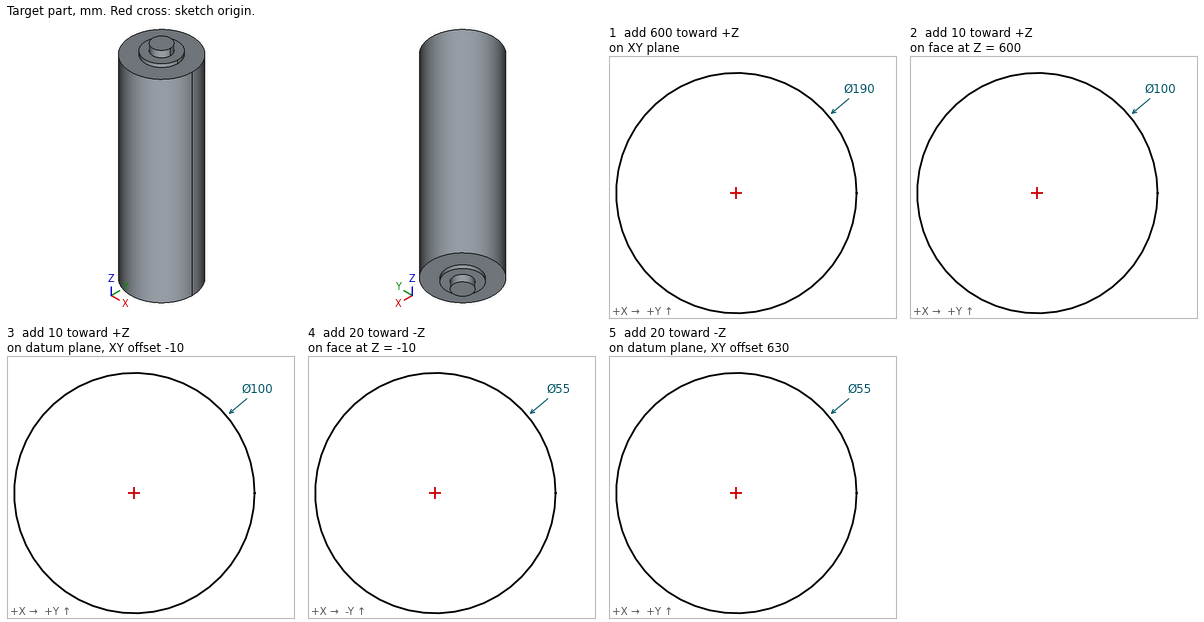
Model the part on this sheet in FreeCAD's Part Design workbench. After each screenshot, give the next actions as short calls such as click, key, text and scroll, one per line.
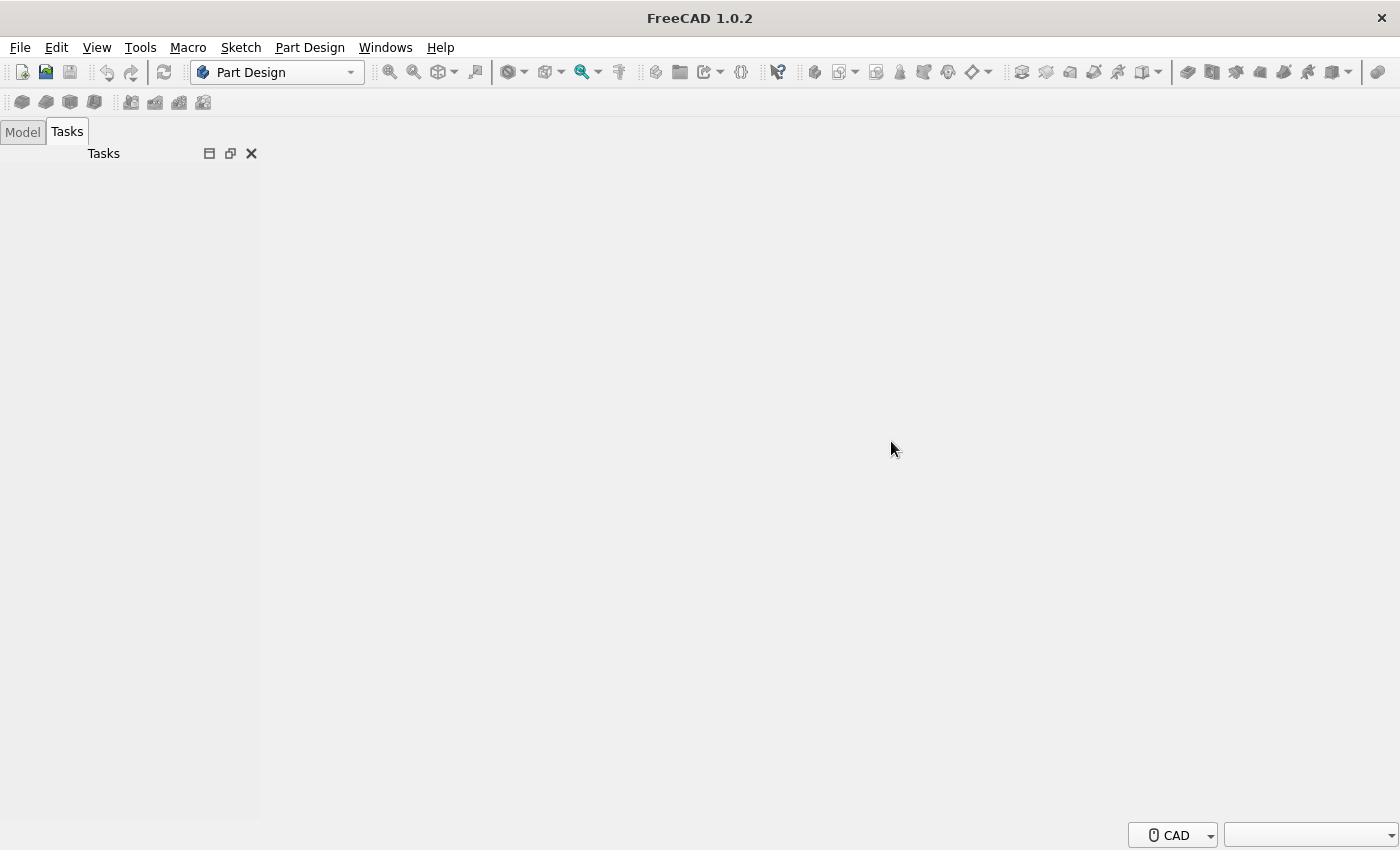
click(22, 72)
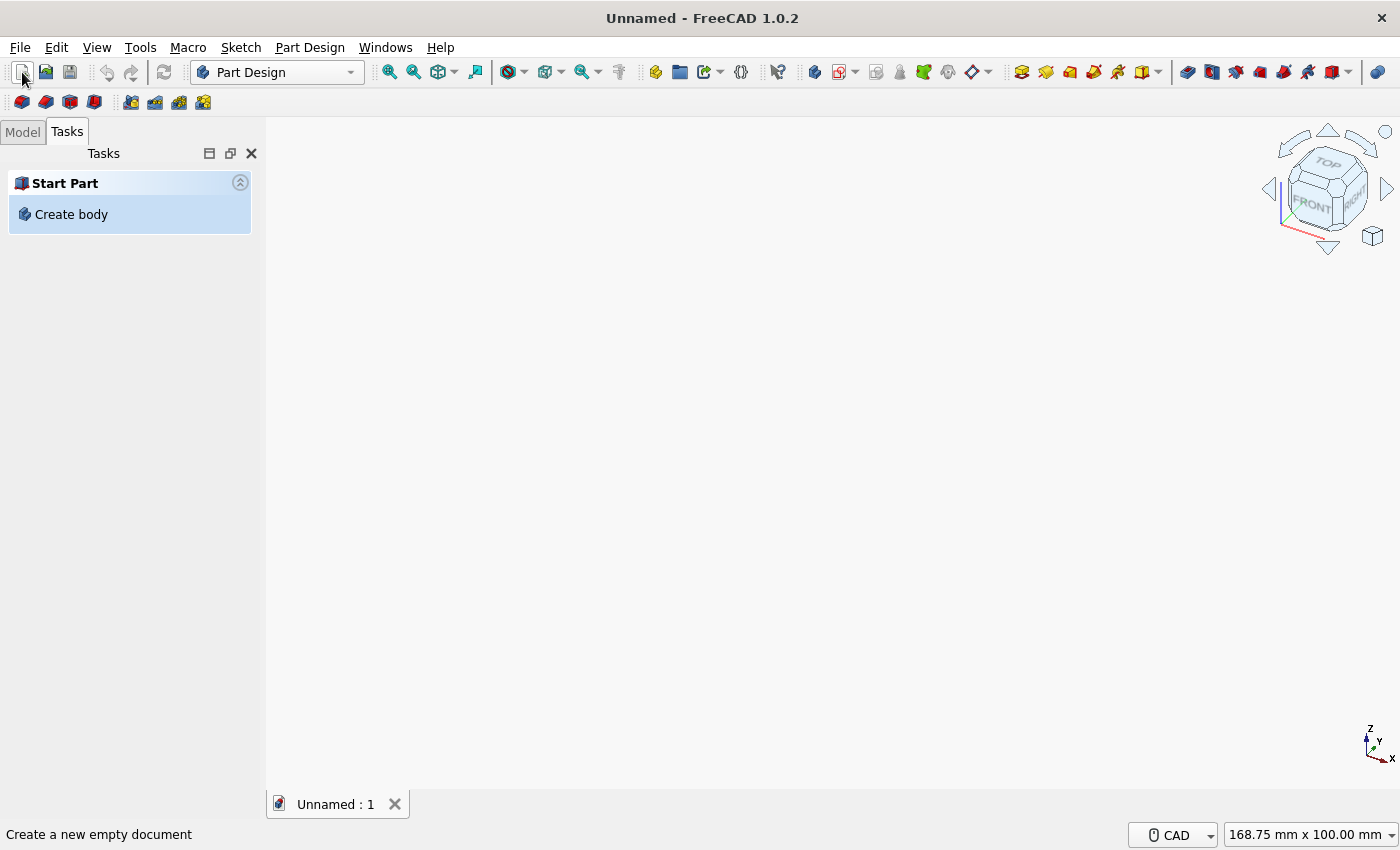
click(840, 72)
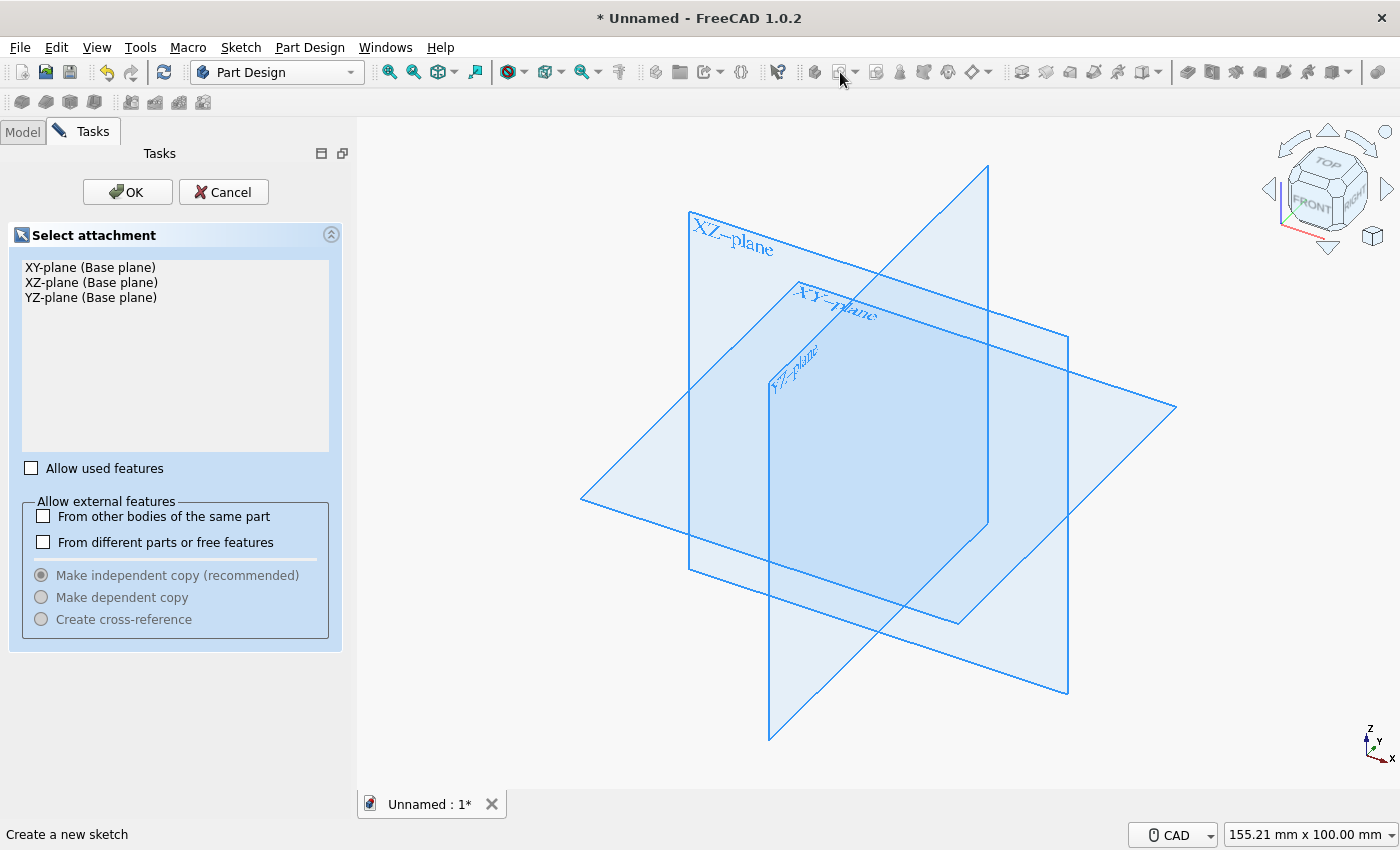
click(82, 268)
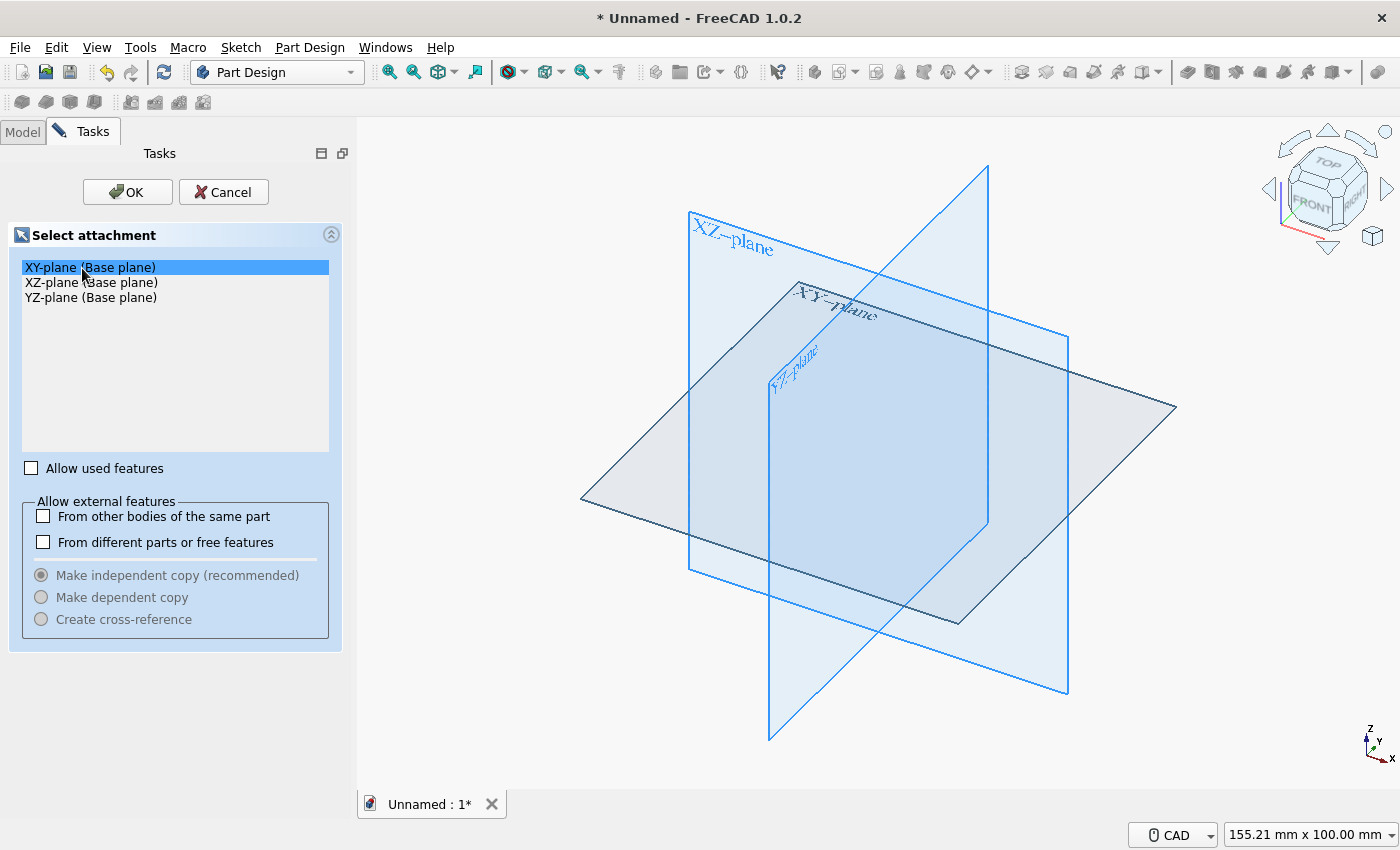
click(128, 192)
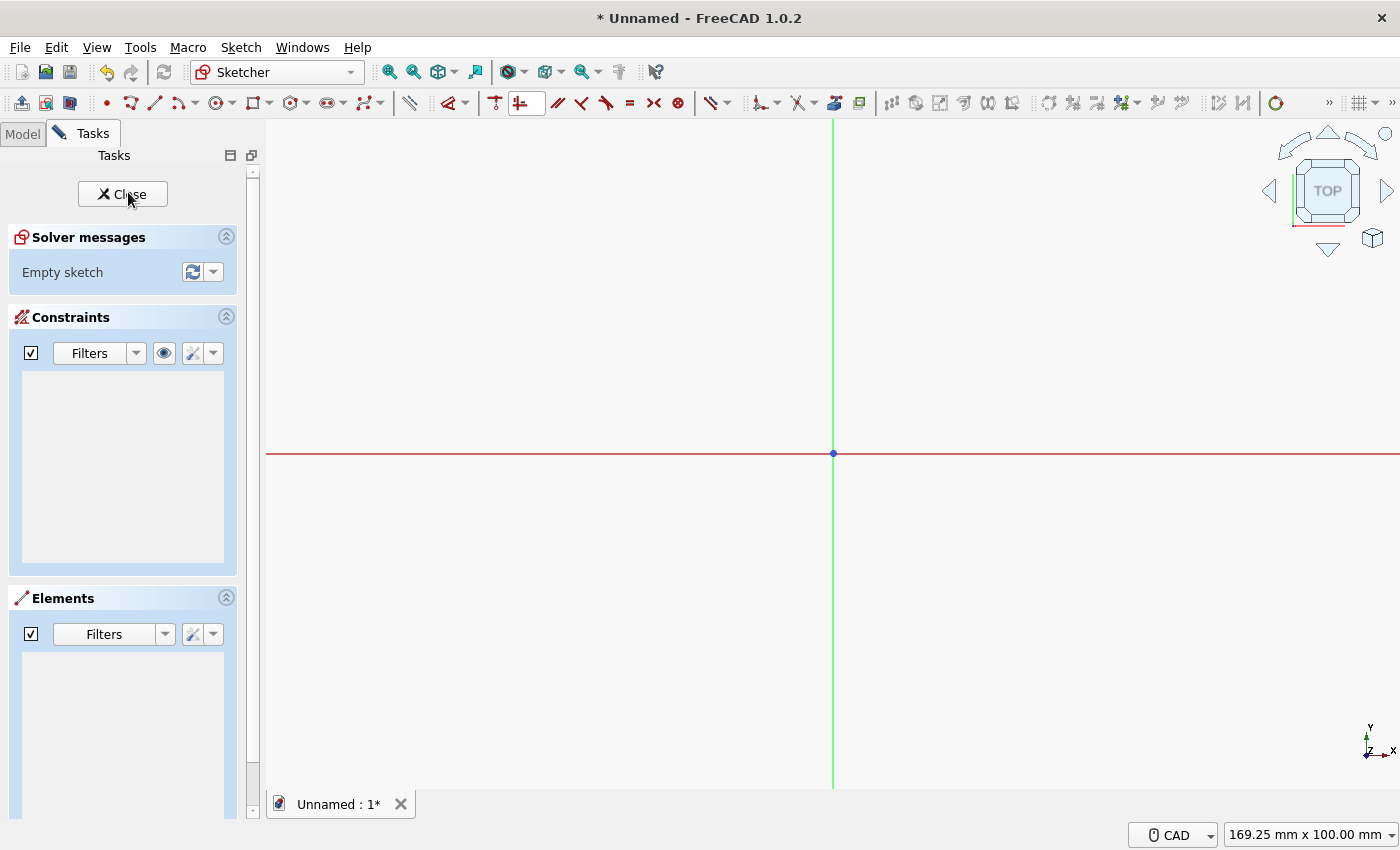
scroll(725, 454, down, 5)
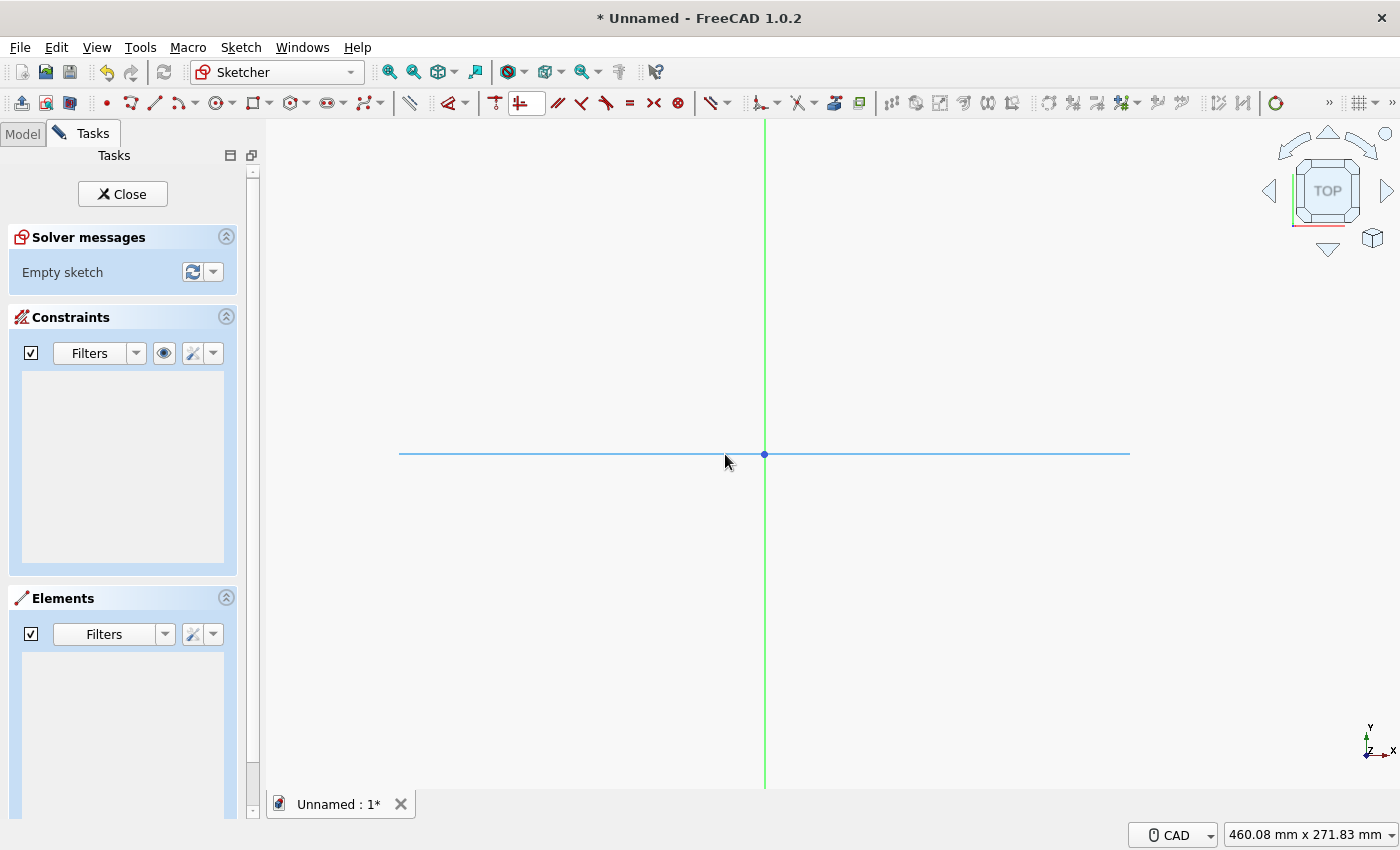
key(g)
key(c)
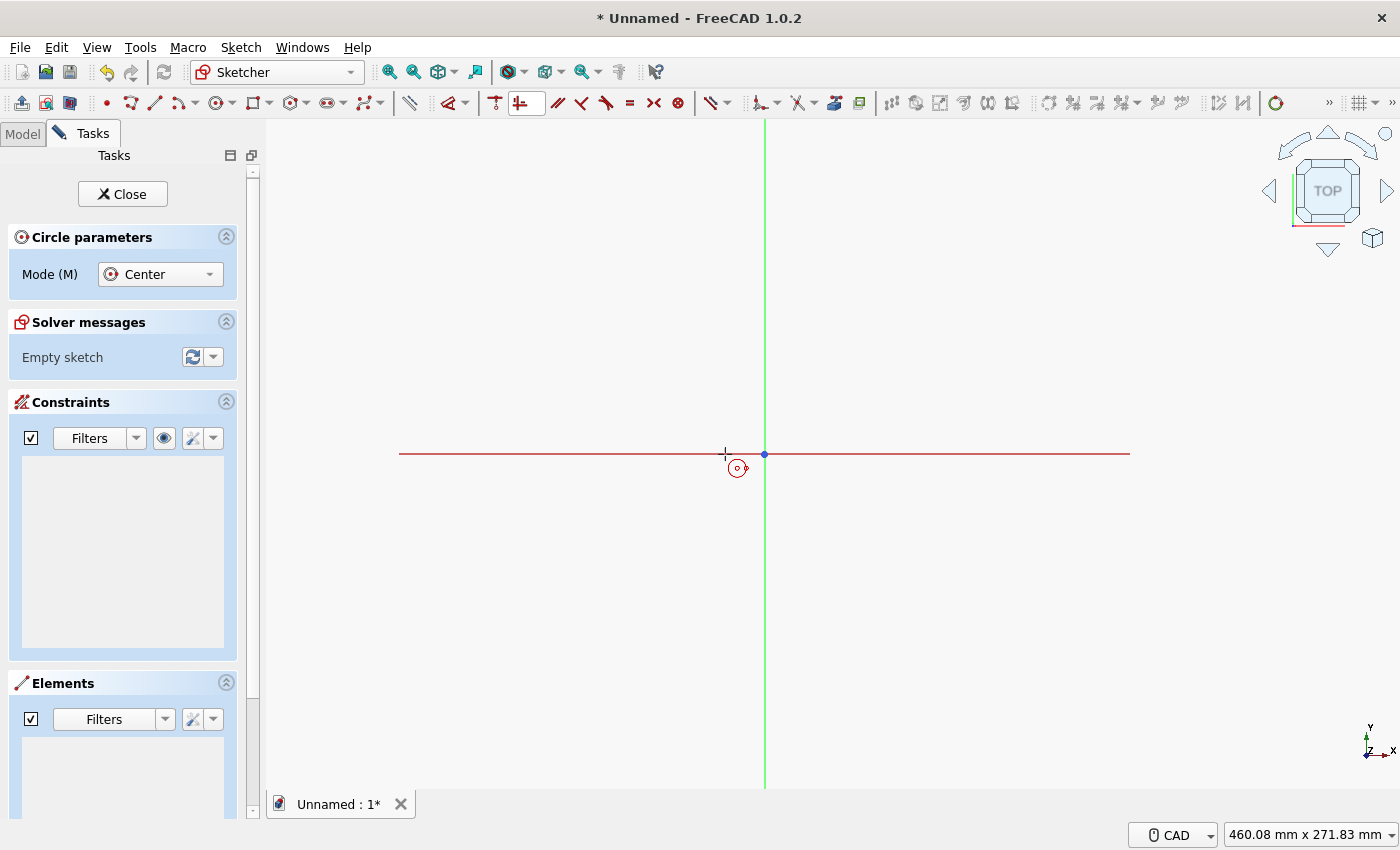
click(765, 454)
click(931, 289)
key(Escape)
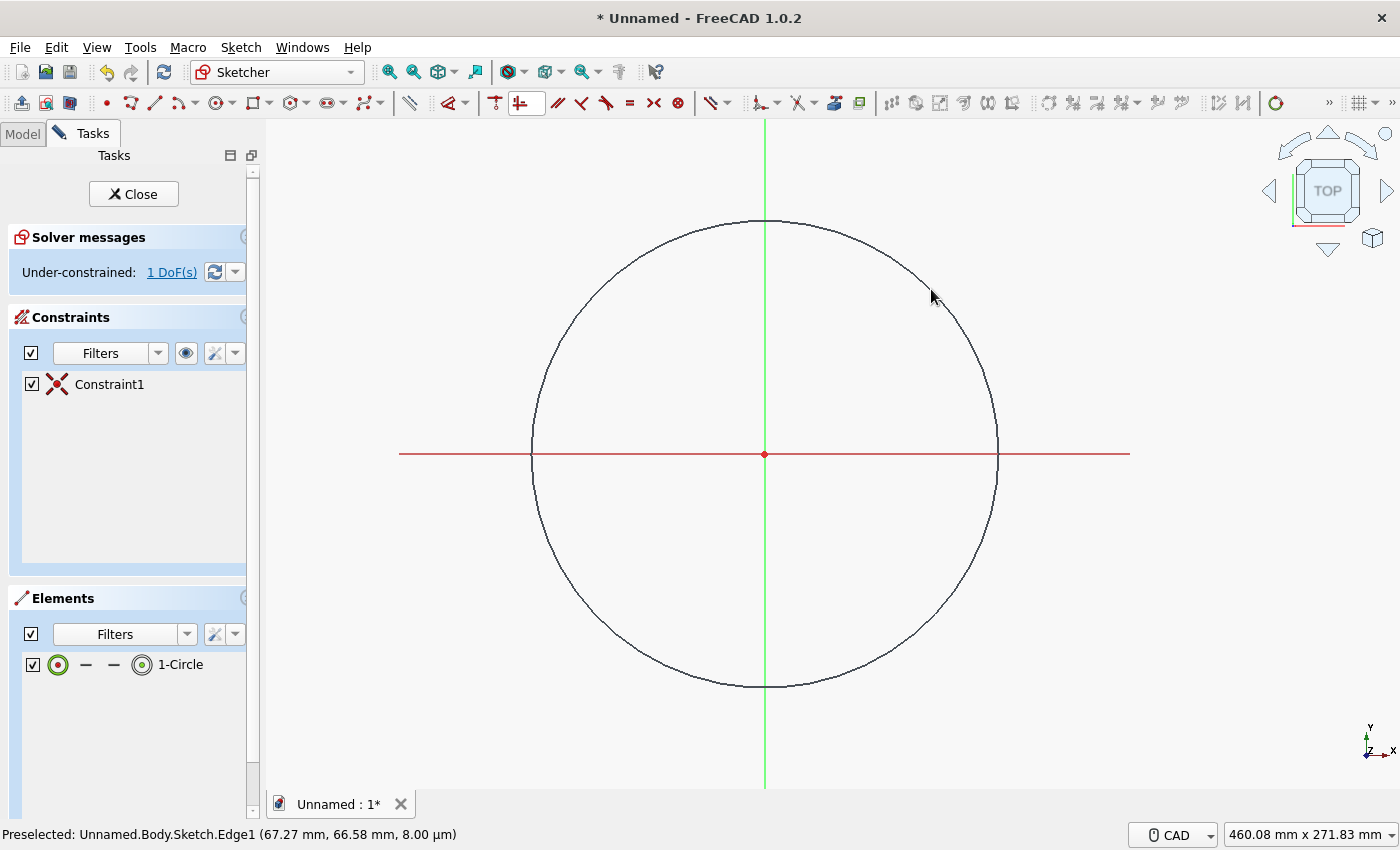
click(448, 104)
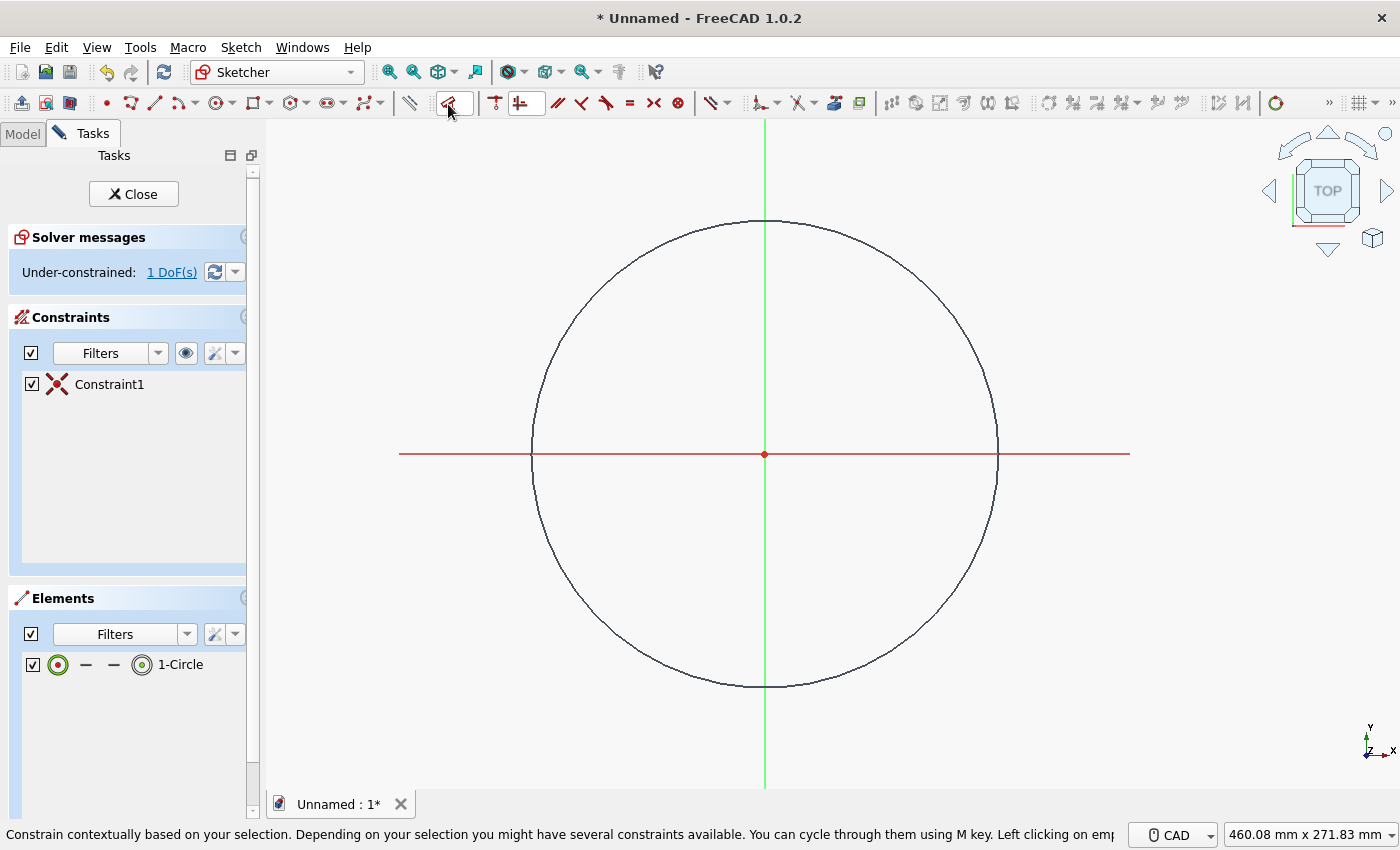
click(930, 289)
click(953, 266)